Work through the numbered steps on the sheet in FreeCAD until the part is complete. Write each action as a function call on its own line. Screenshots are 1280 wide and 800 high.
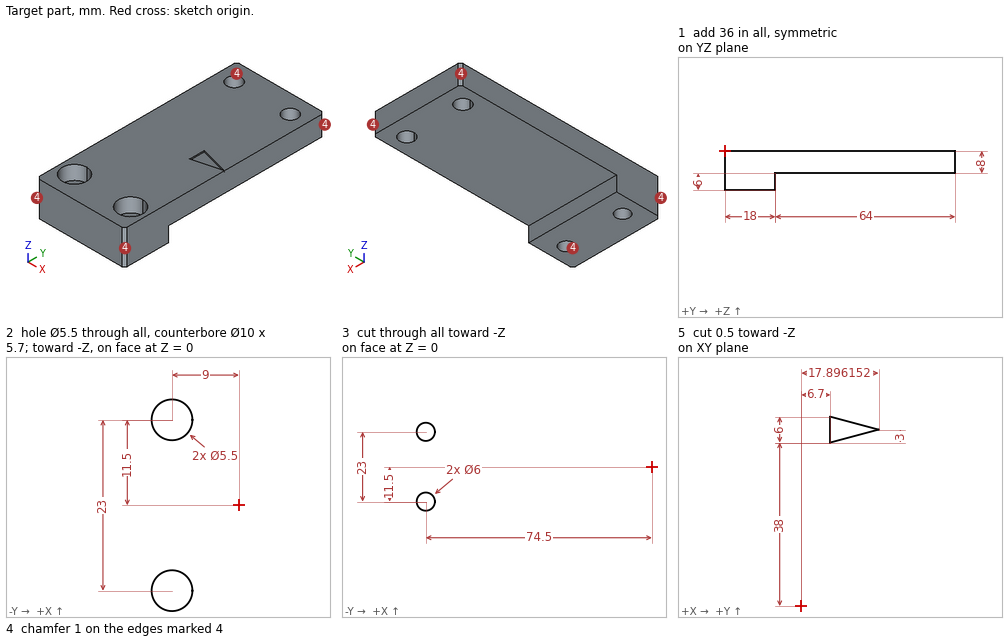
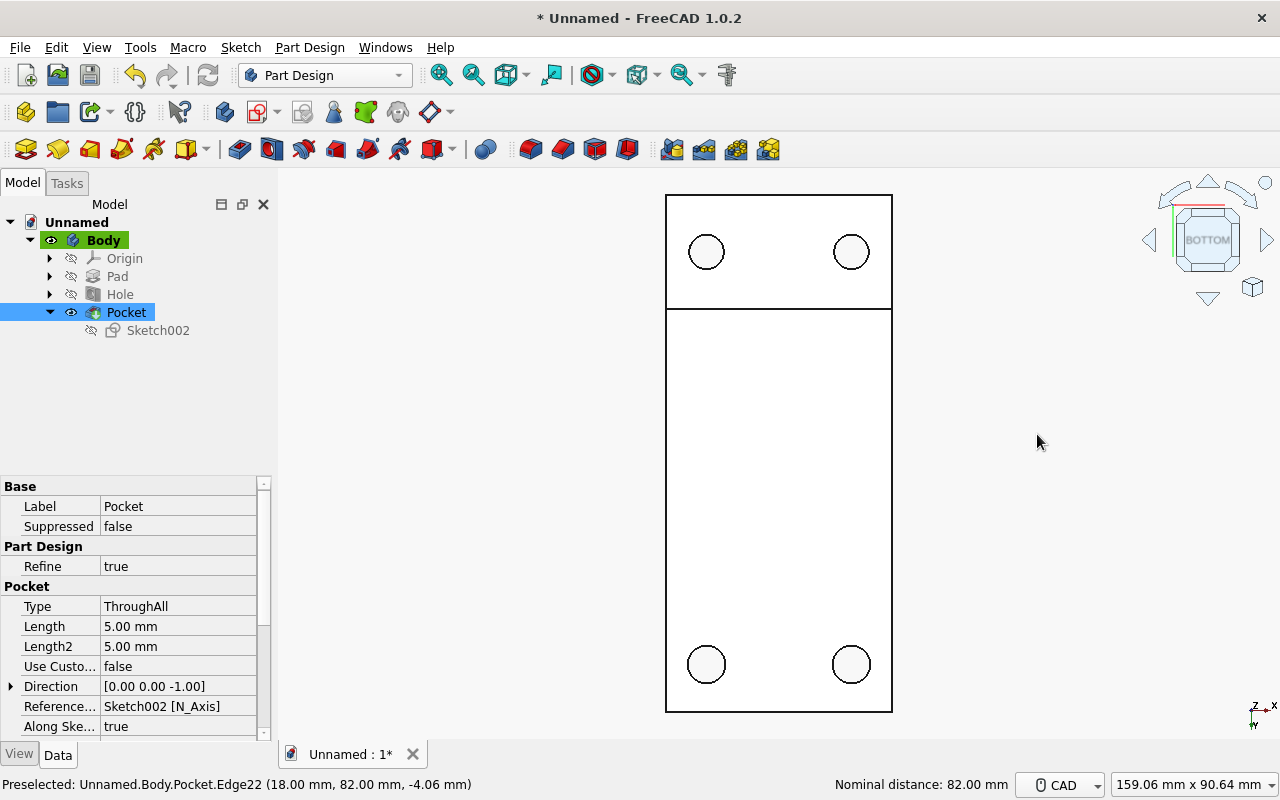
key(4)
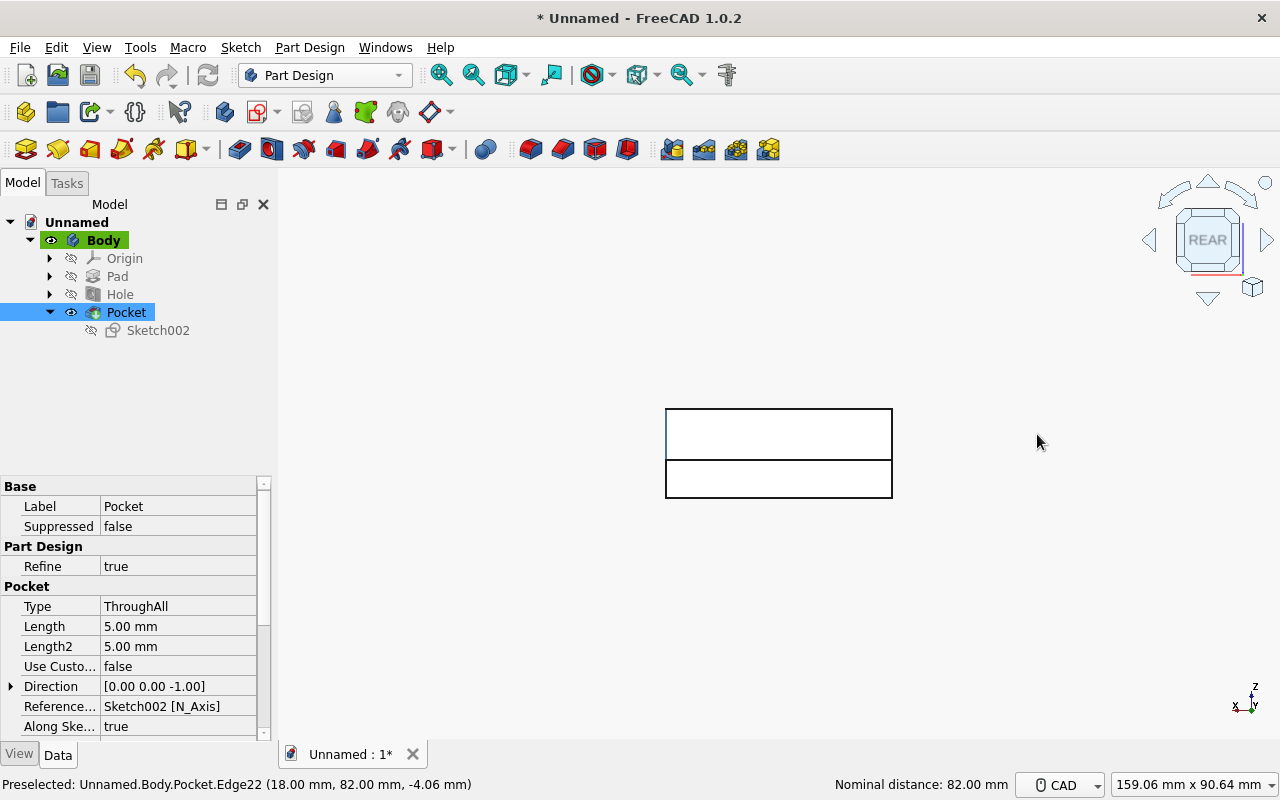
key(v)
key(f)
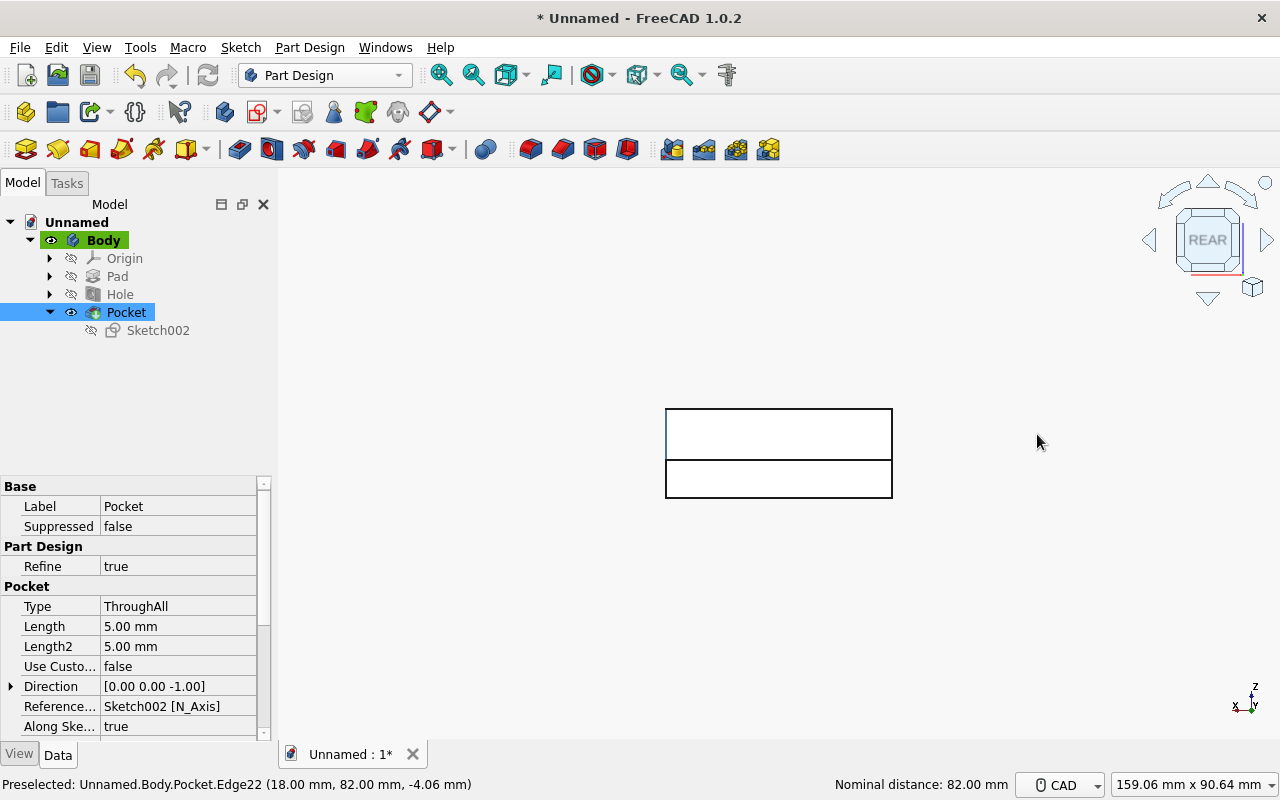
click(892, 434, ctrl)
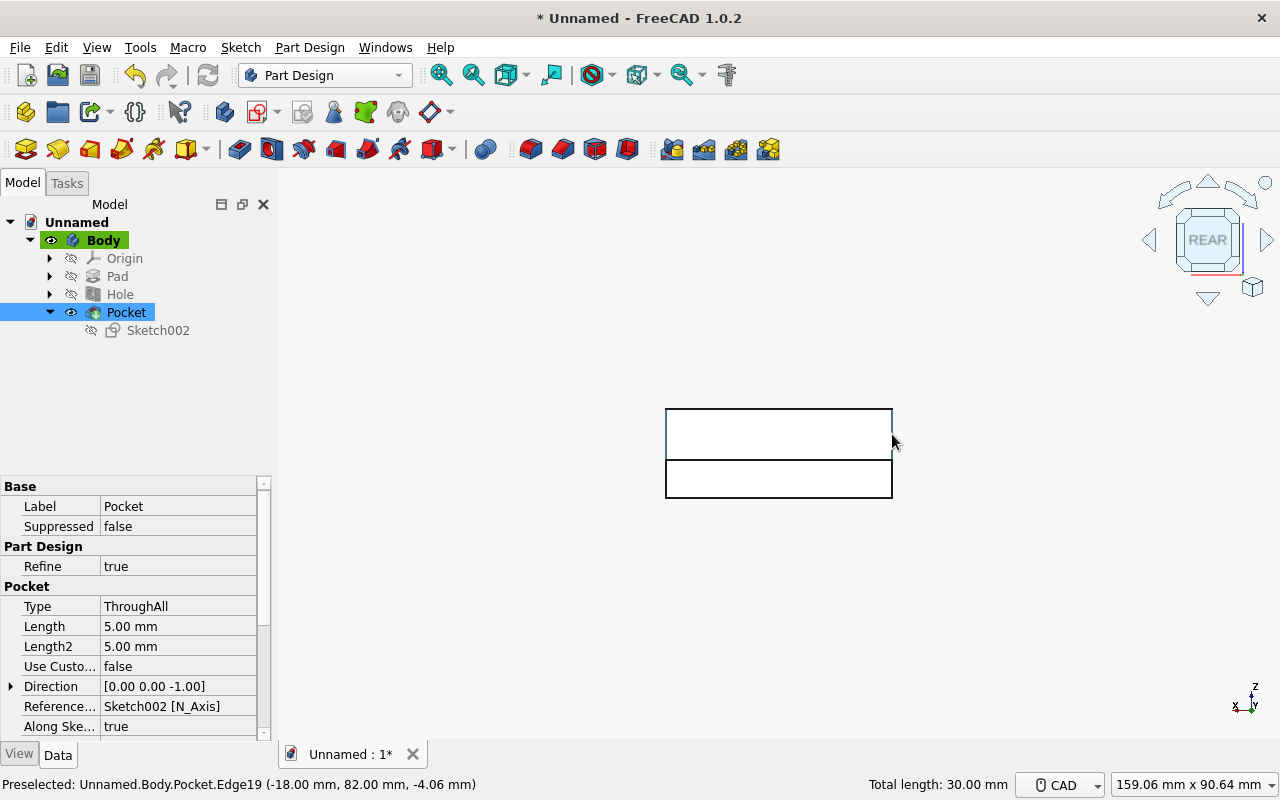
key(6)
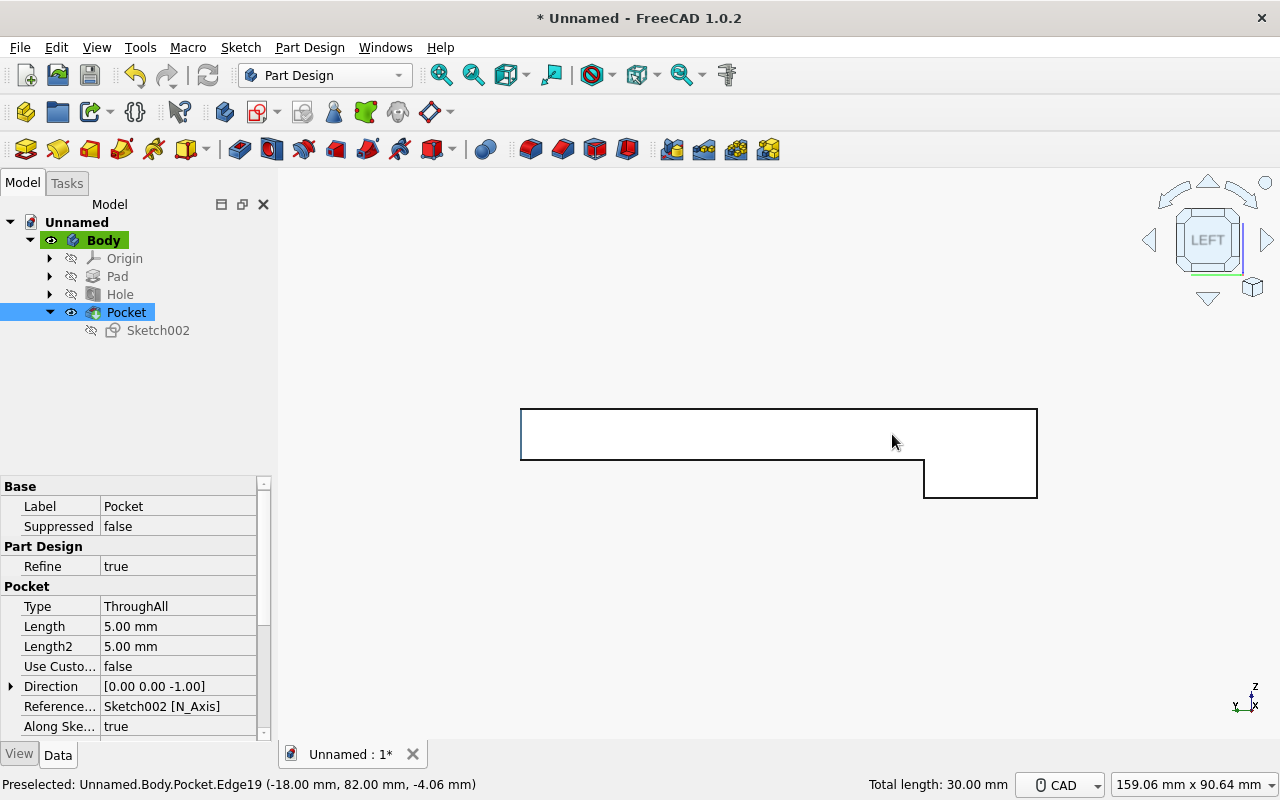
click(1037, 452, ctrl)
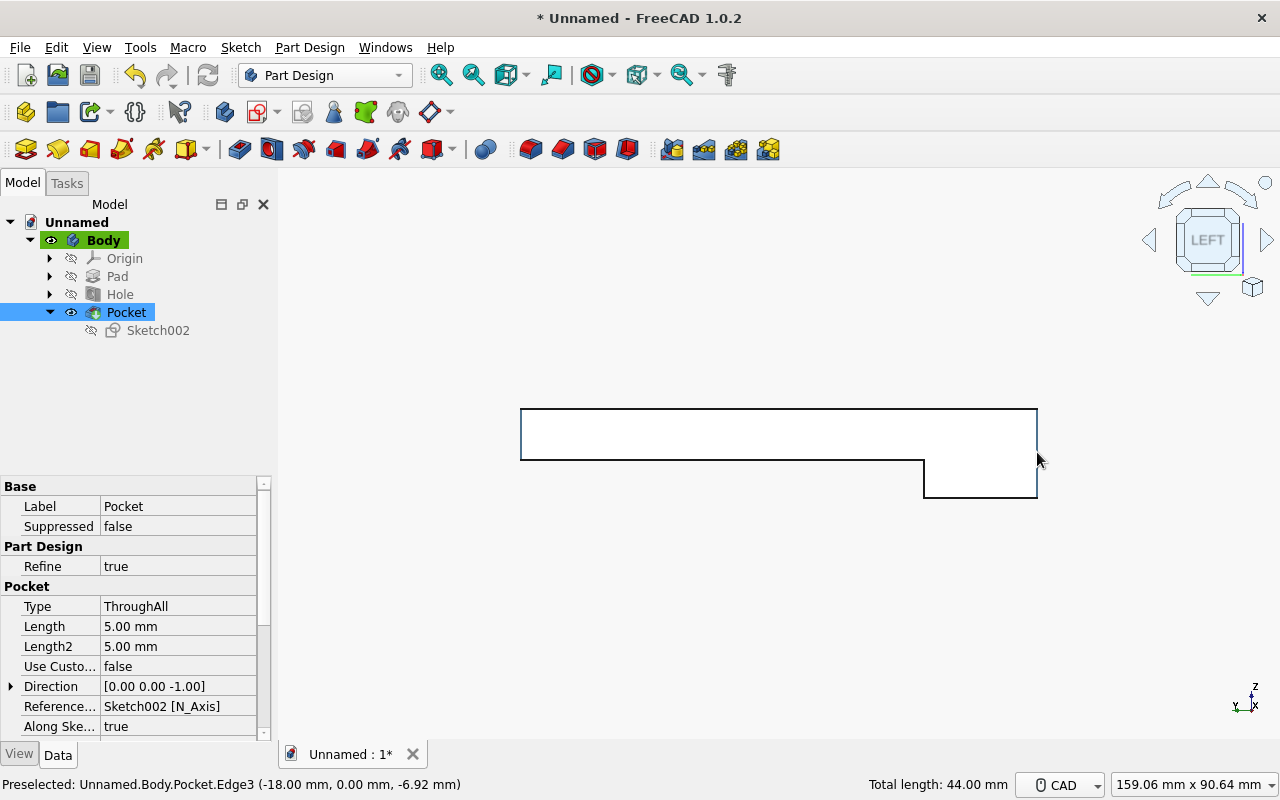
click(564, 150)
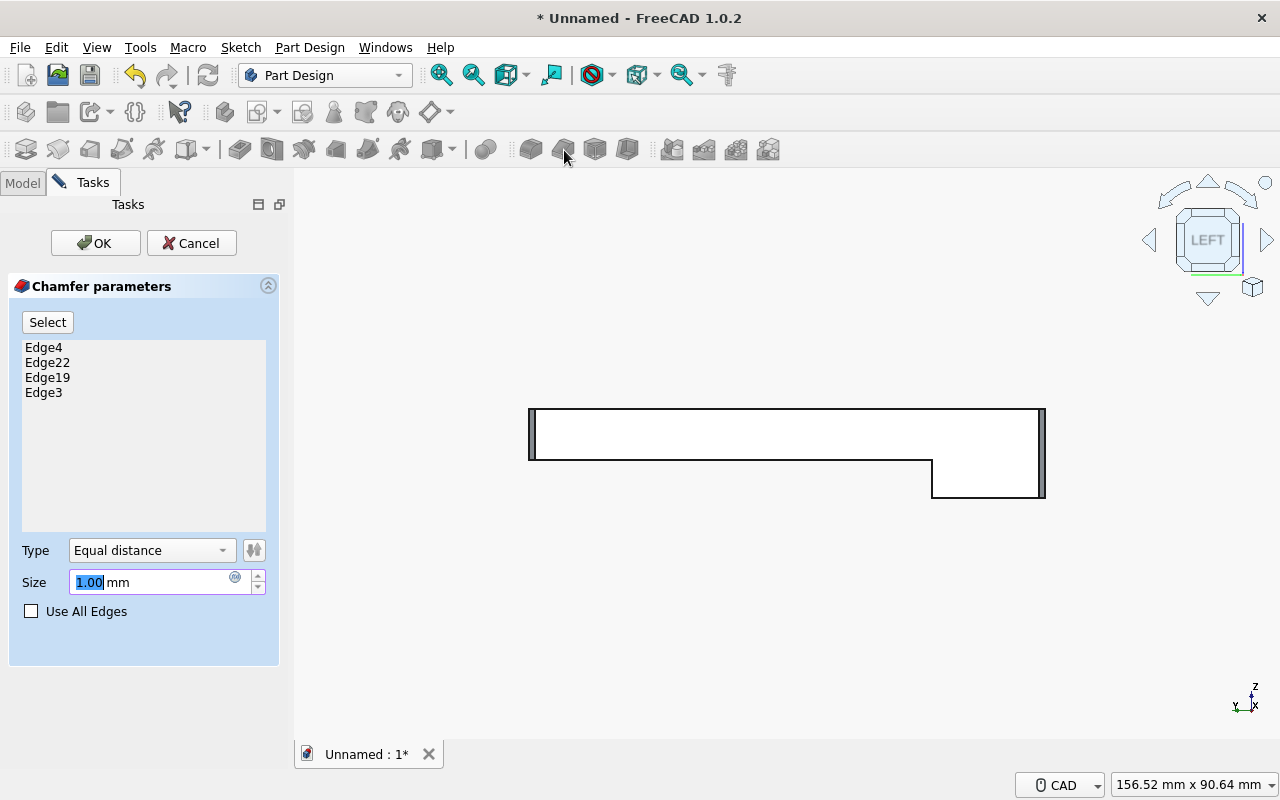
text(1)
key(Tab)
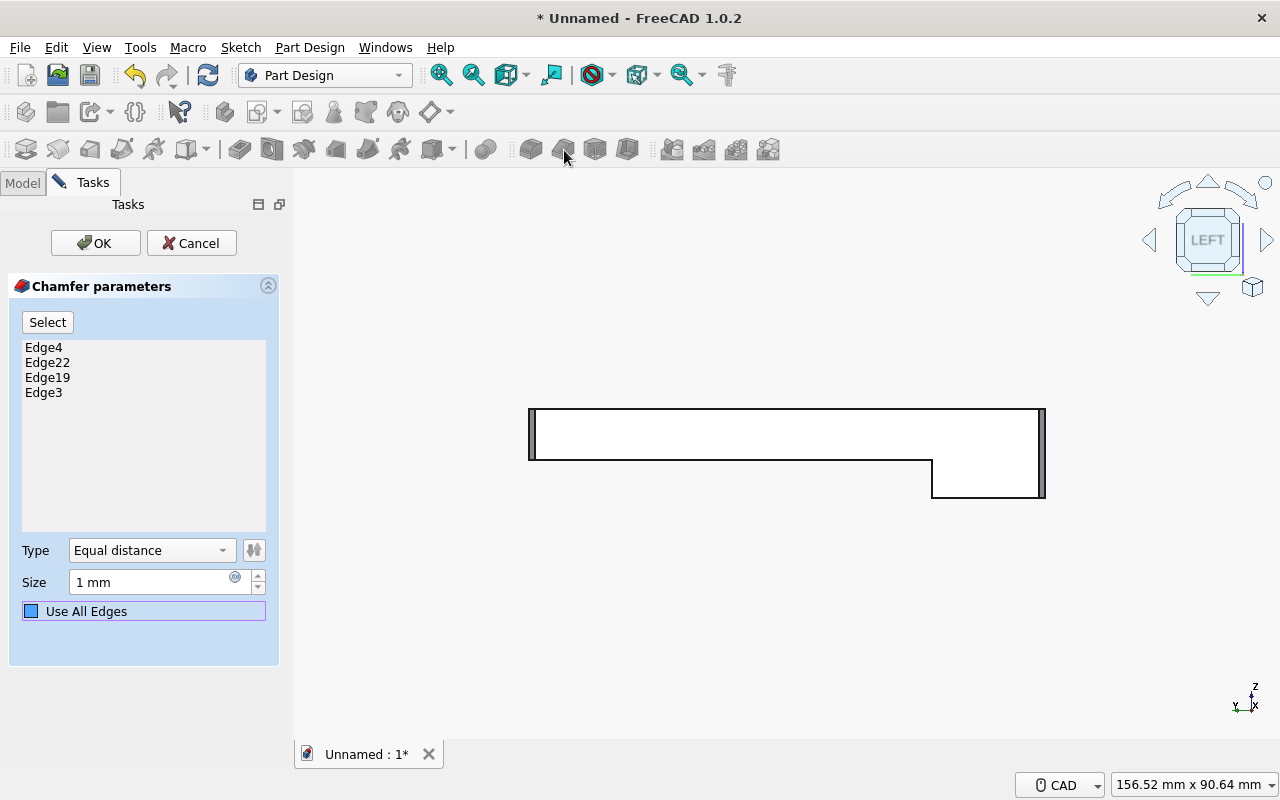
click(96, 243)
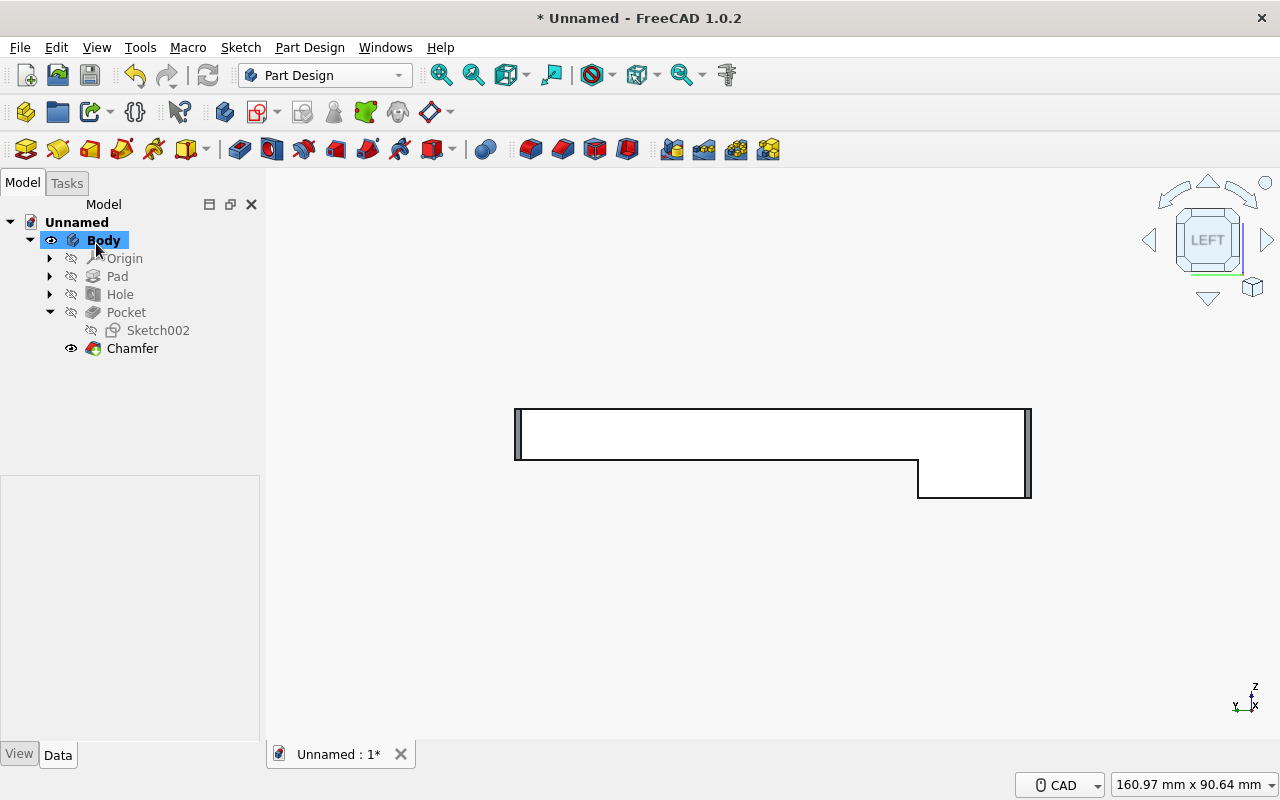
click(258, 112)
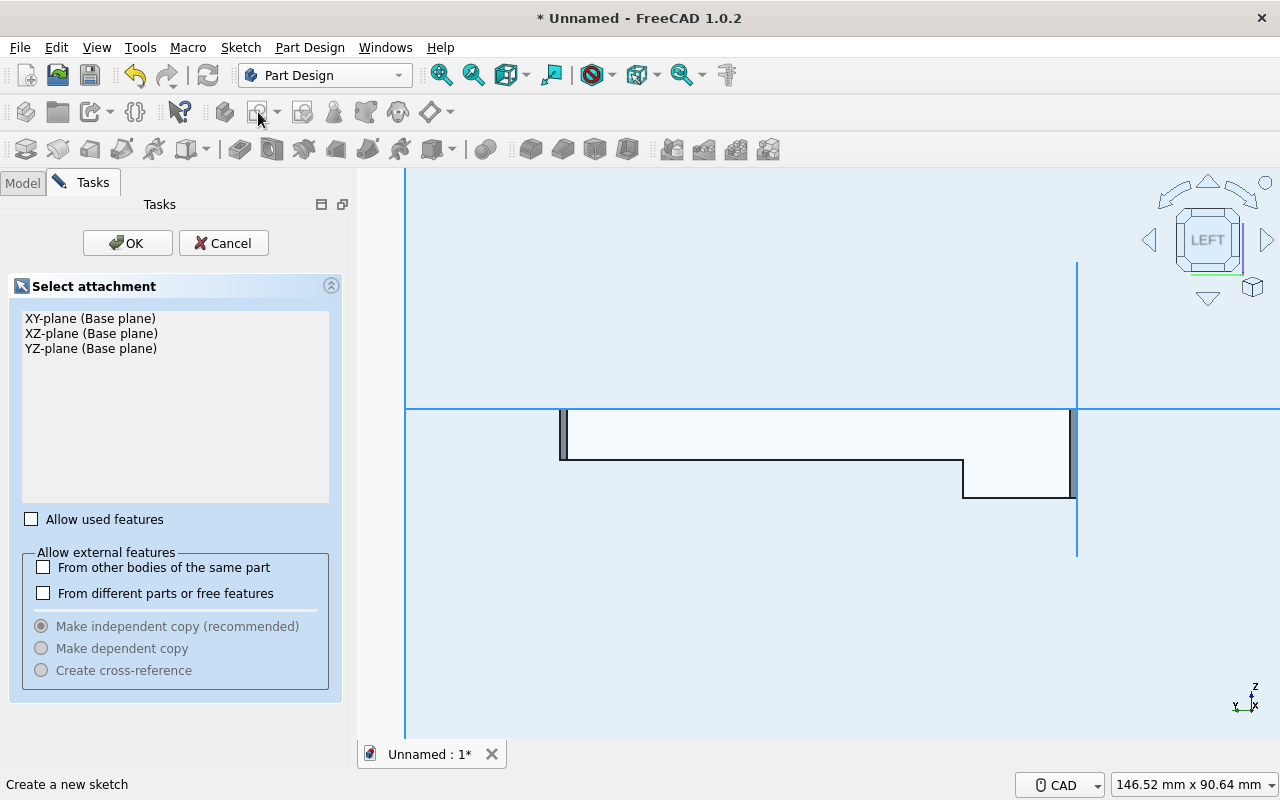
click(82, 318)